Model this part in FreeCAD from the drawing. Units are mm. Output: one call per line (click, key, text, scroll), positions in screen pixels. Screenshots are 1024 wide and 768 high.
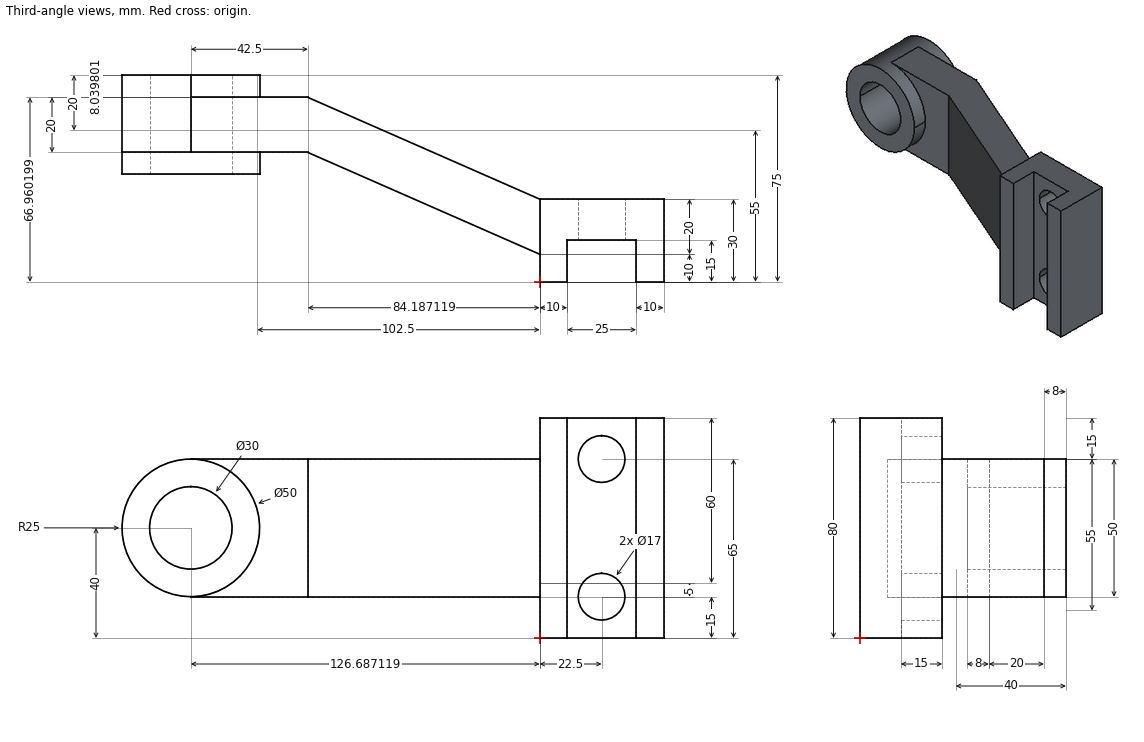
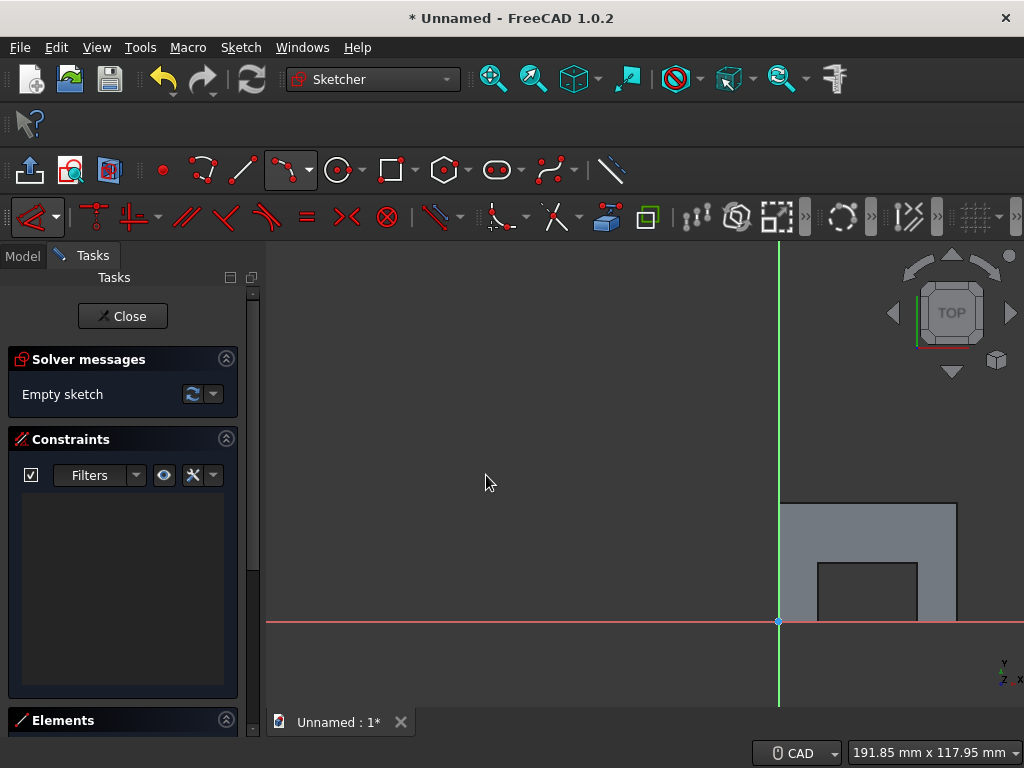
key(g)
key(m)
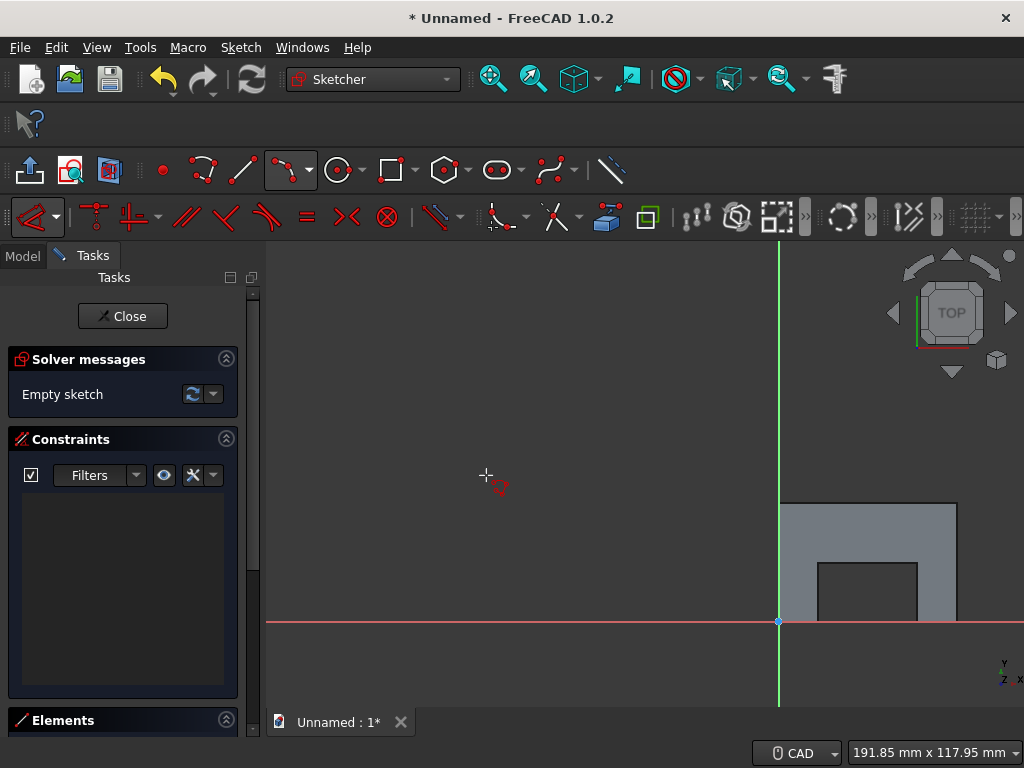
click(779, 582)
click(770, 503)
click(374, 326)
click(374, 405)
click(779, 583)
key(Escape)
key(Escape)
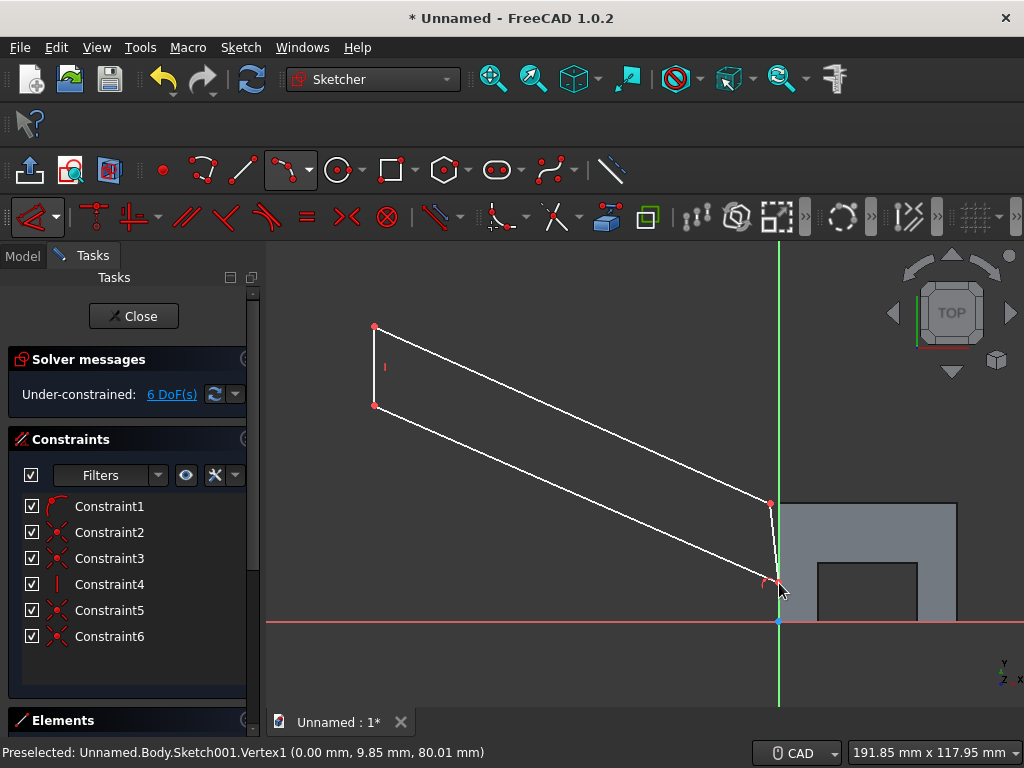
click(776, 559)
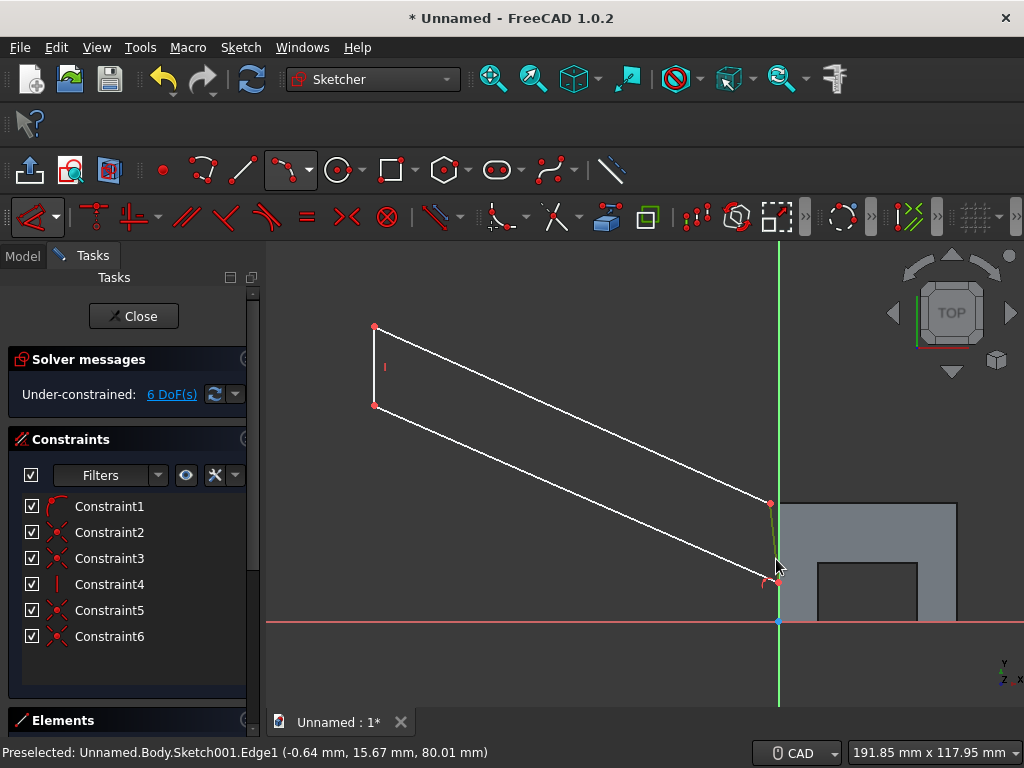
key(v)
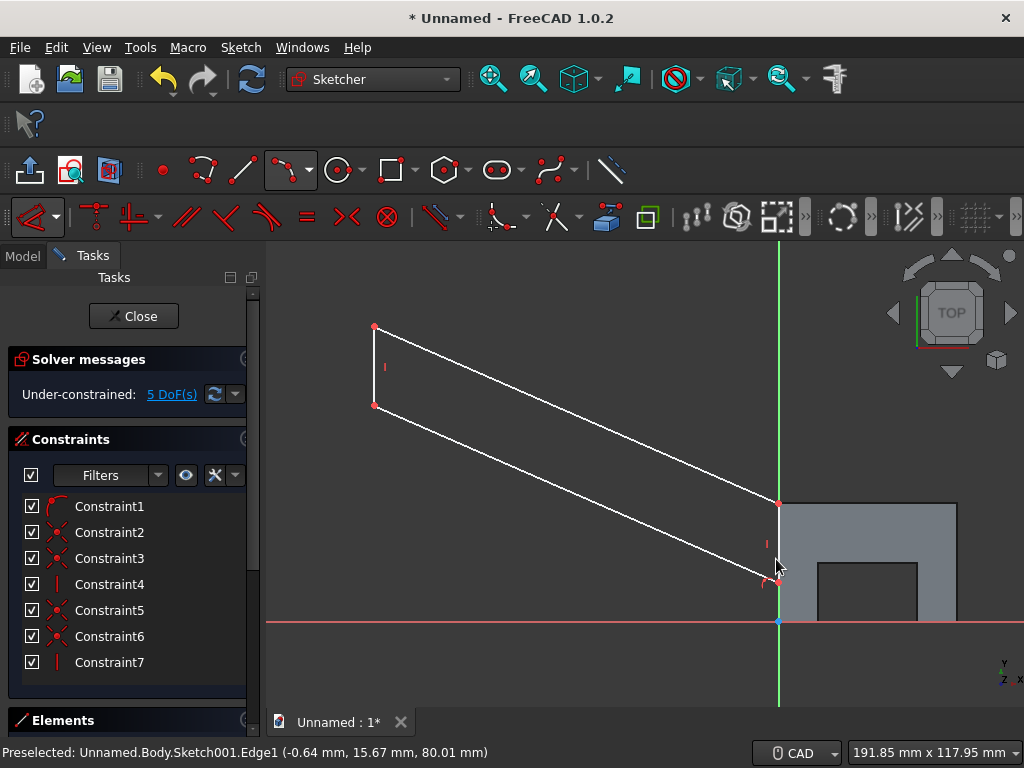
click(779, 559)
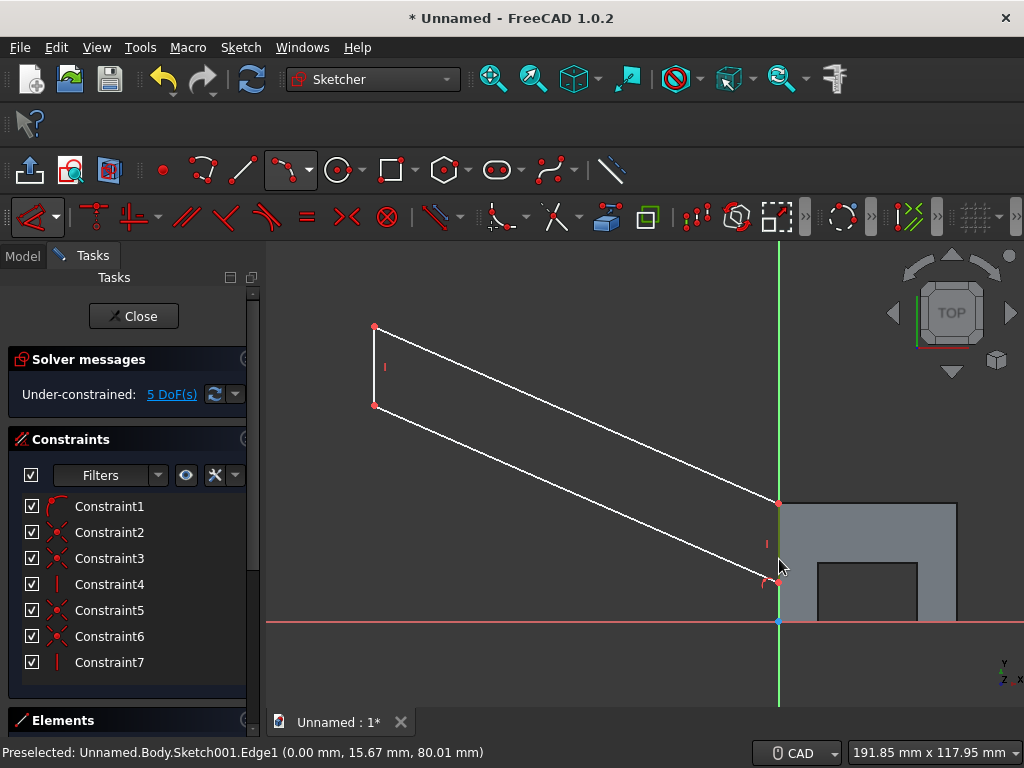
key(i)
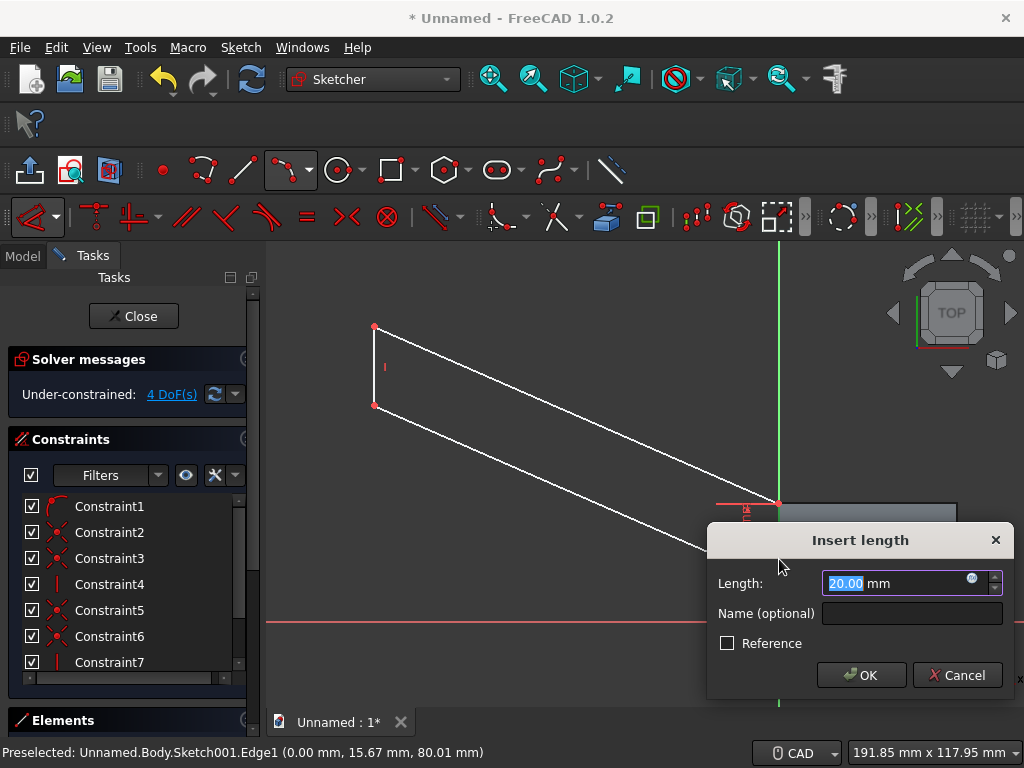
text(20)
key(Return)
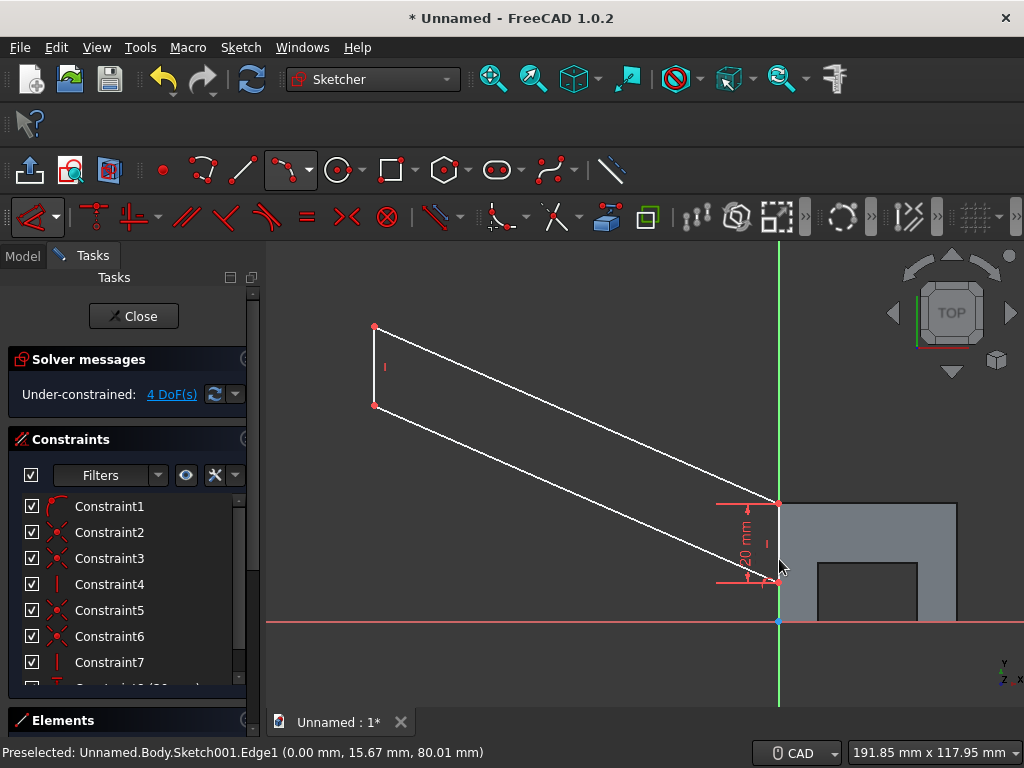
click(374, 351)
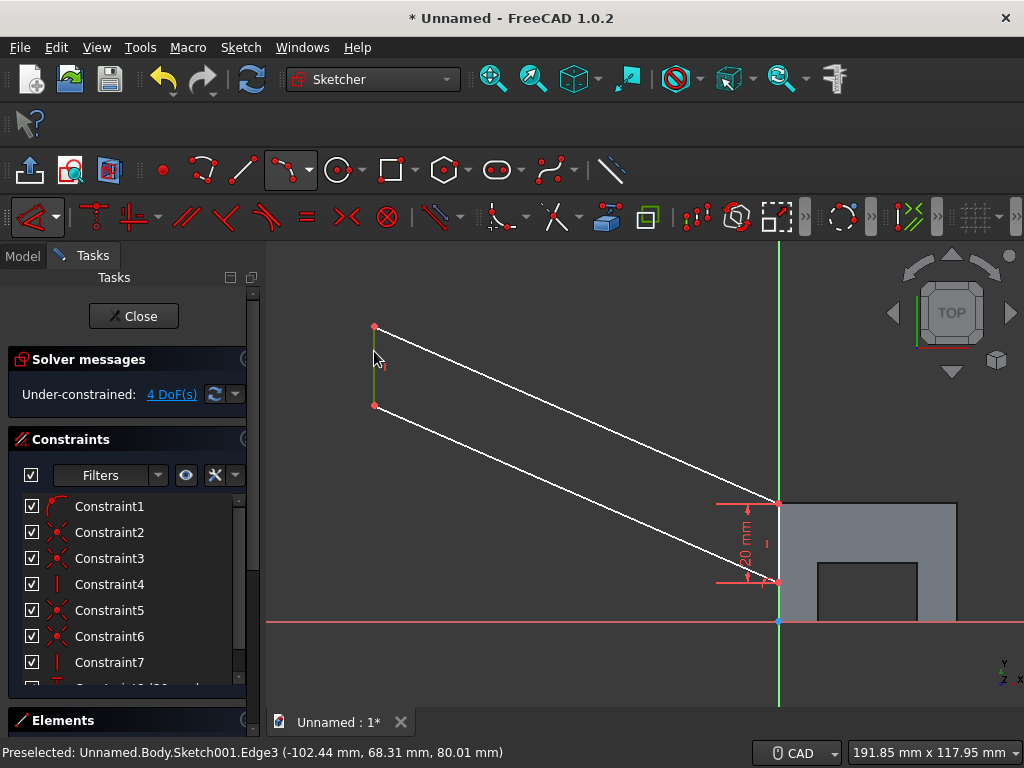
key(i)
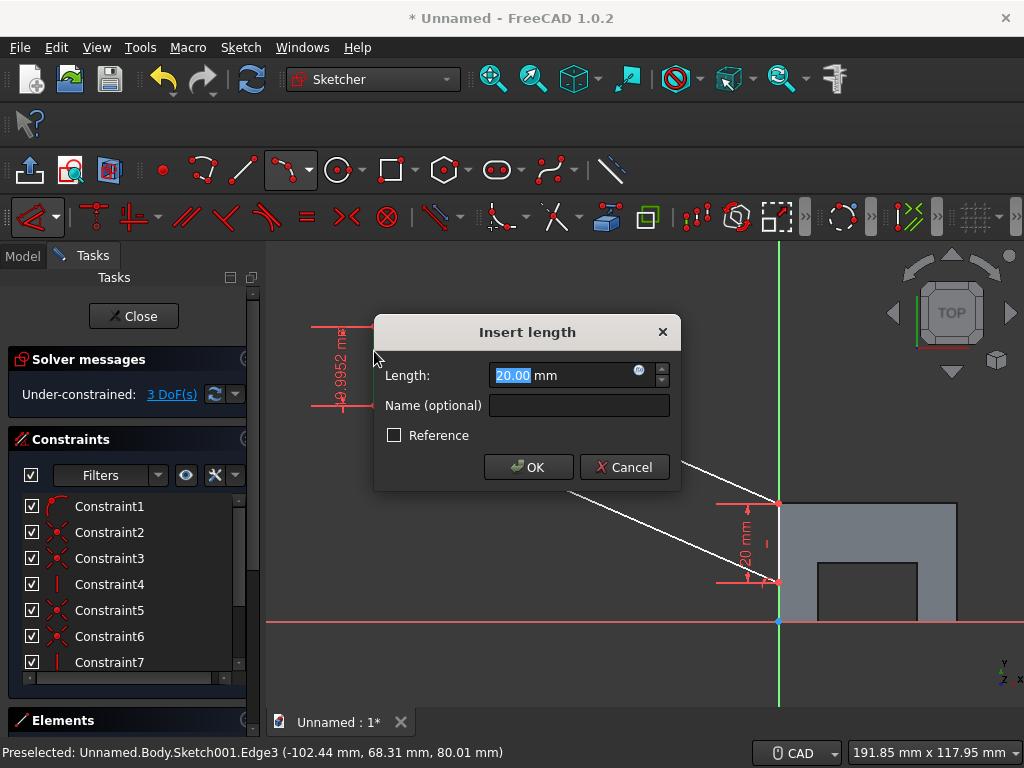
text(20)
key(Return)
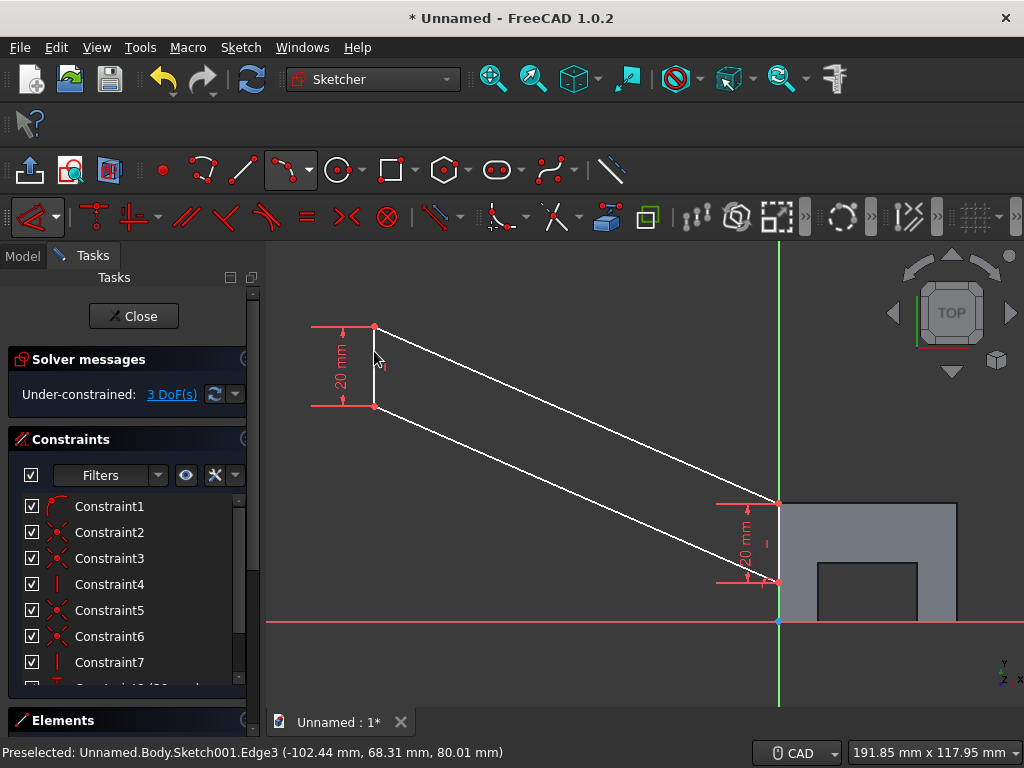
click(779, 583)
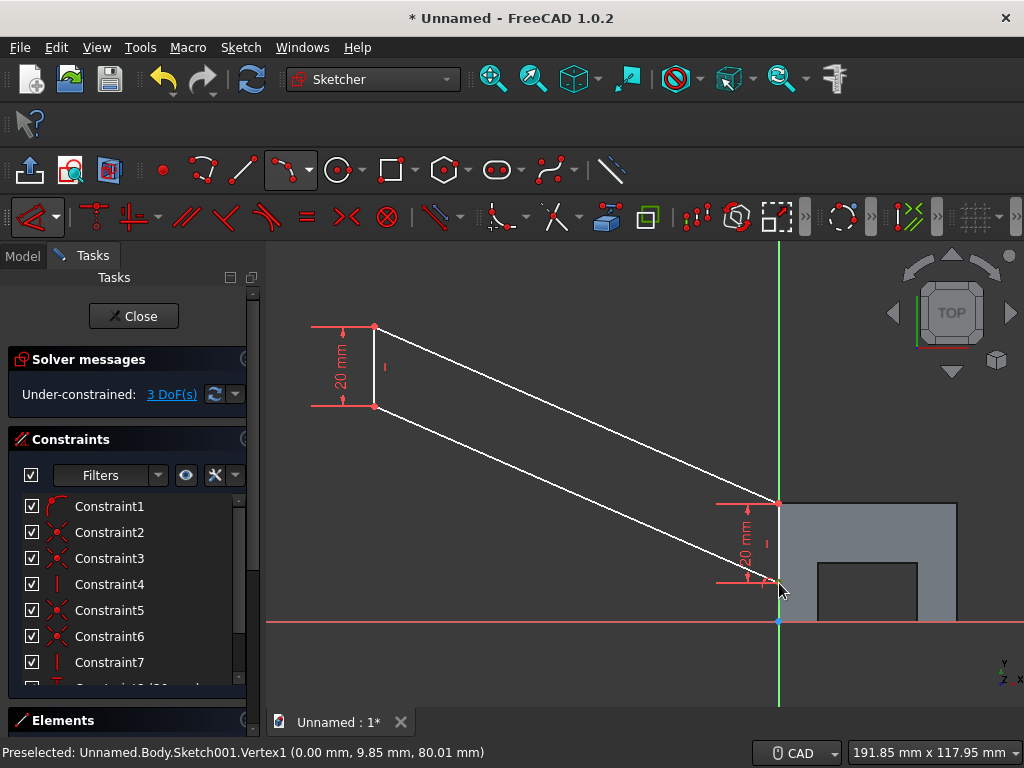
key(i)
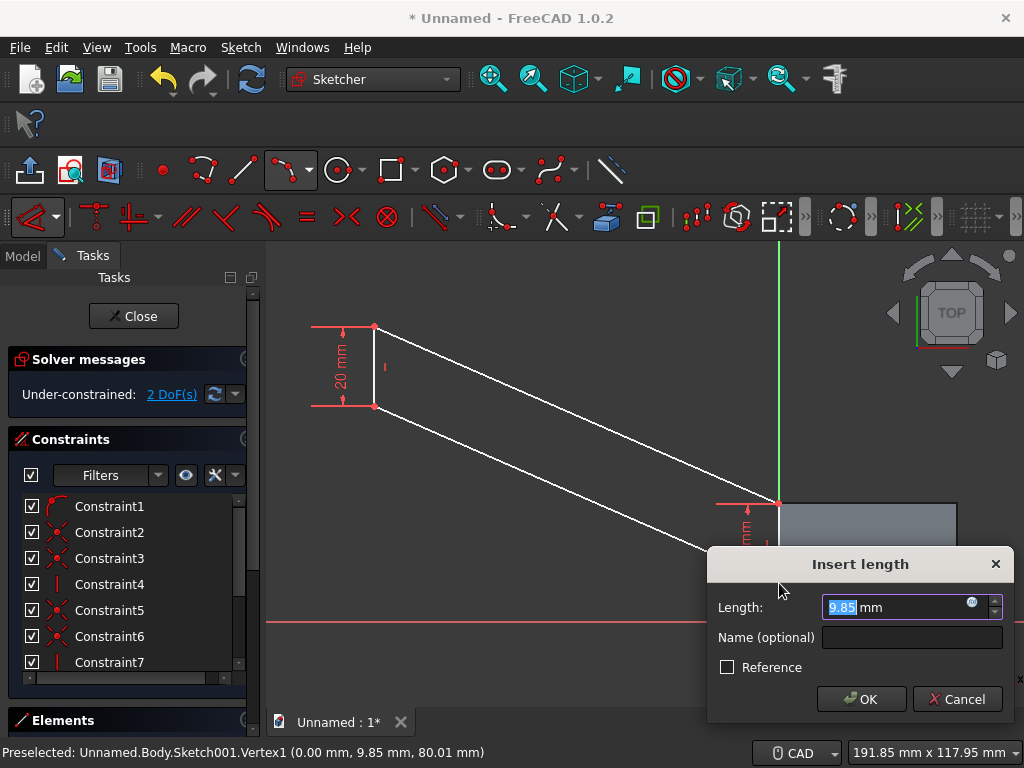
text(10)
key(Return)